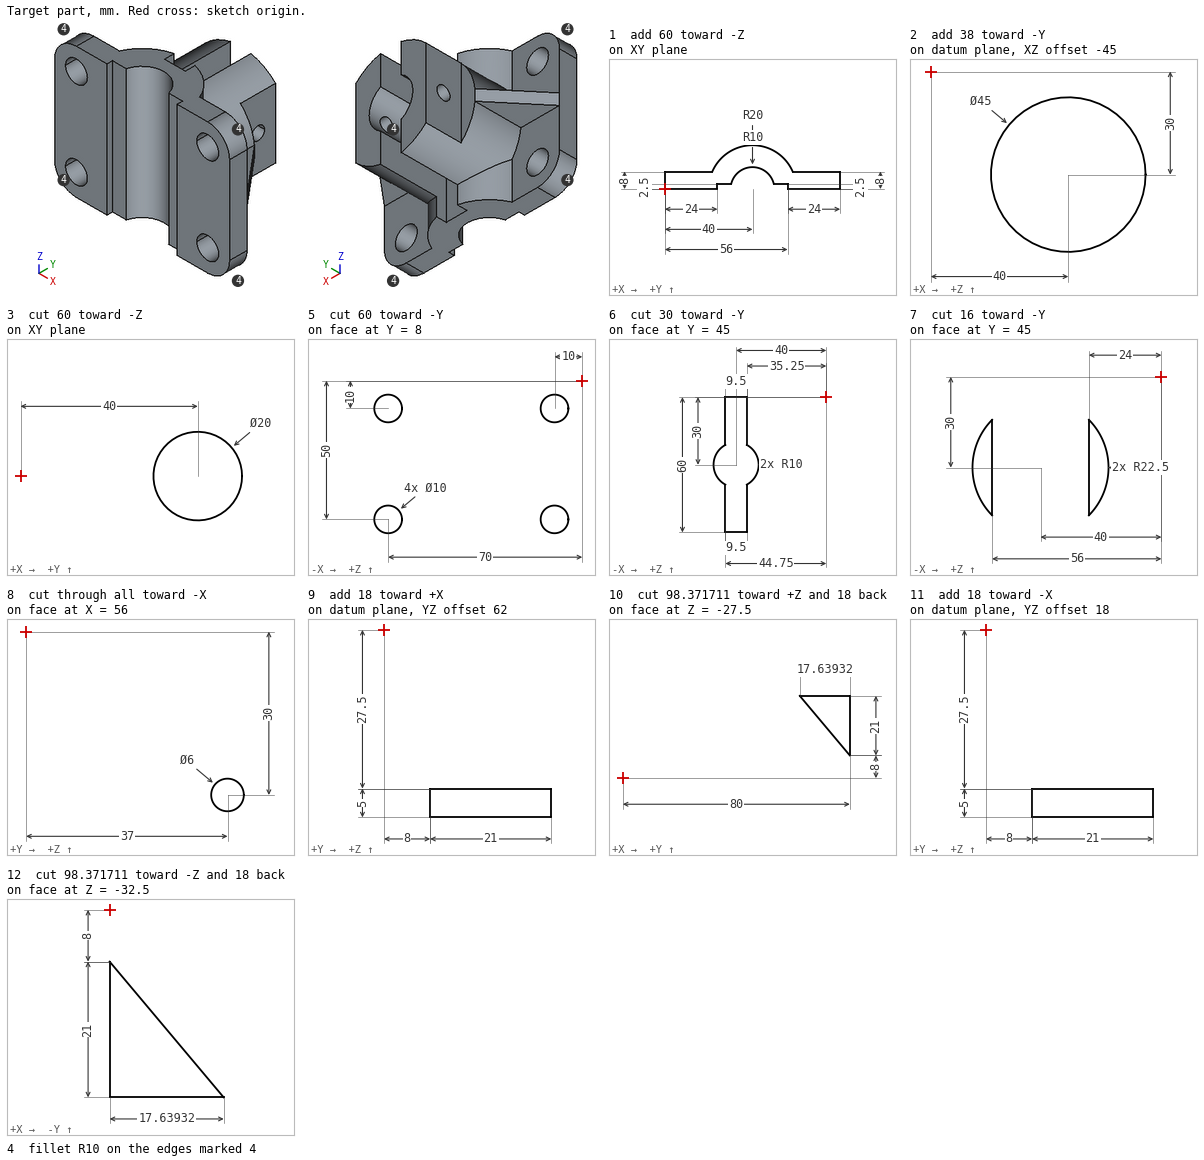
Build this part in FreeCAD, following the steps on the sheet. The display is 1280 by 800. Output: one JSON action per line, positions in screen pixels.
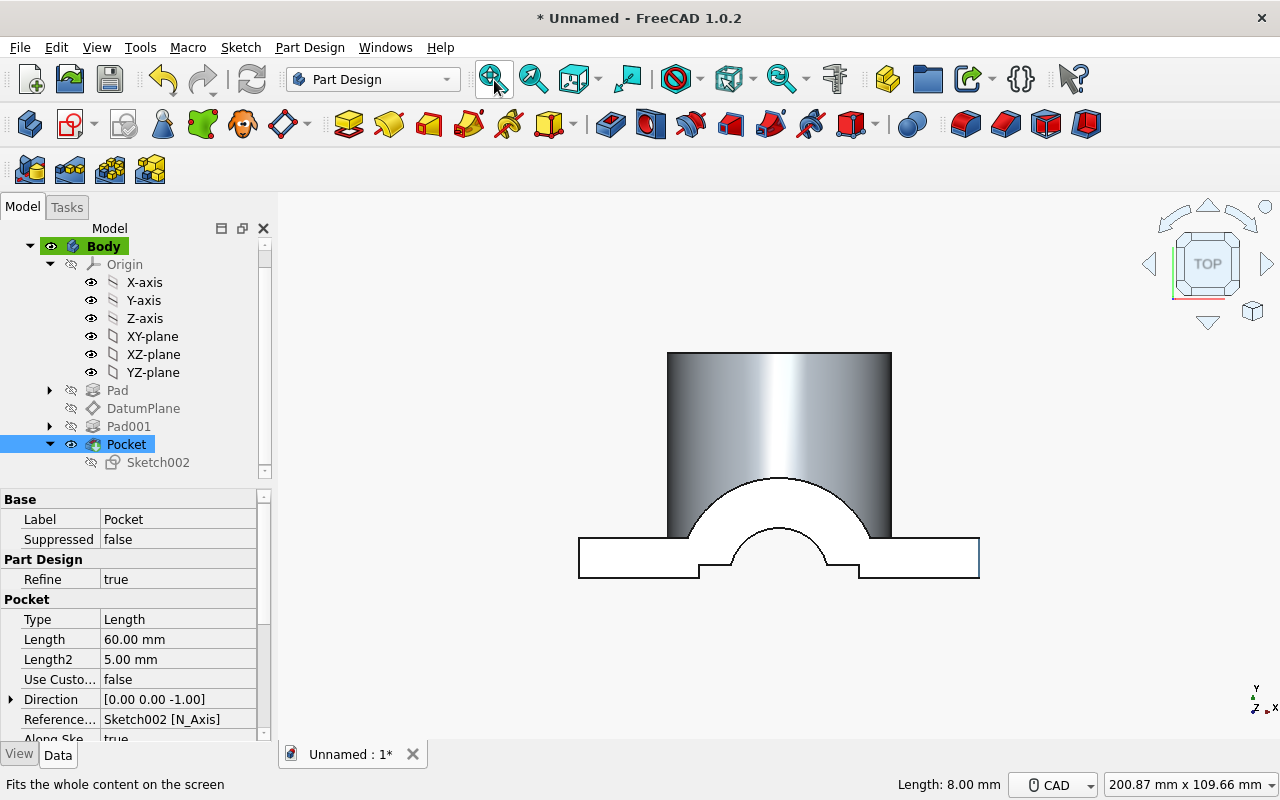
{"action": "left_click", "coordinate": [579, 557], "text": "ctrl"}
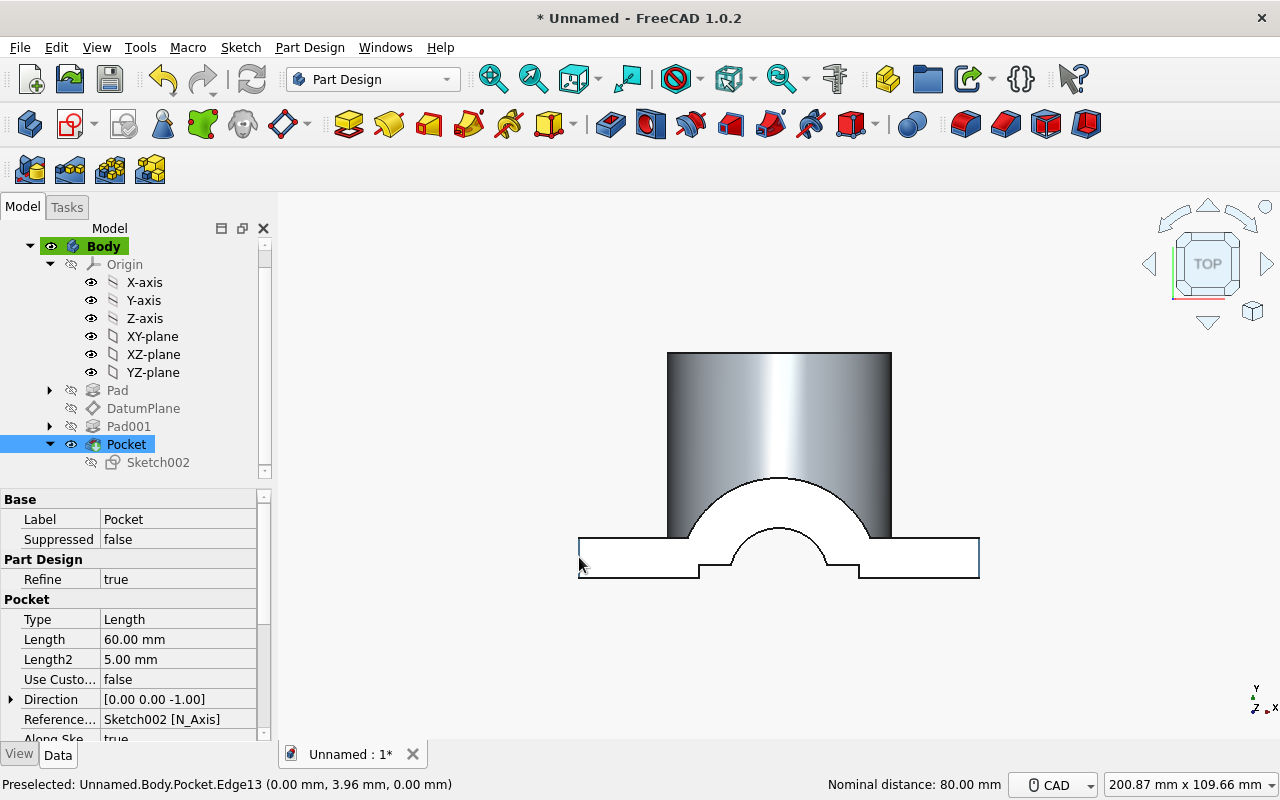
{"action": "key", "text": "1"}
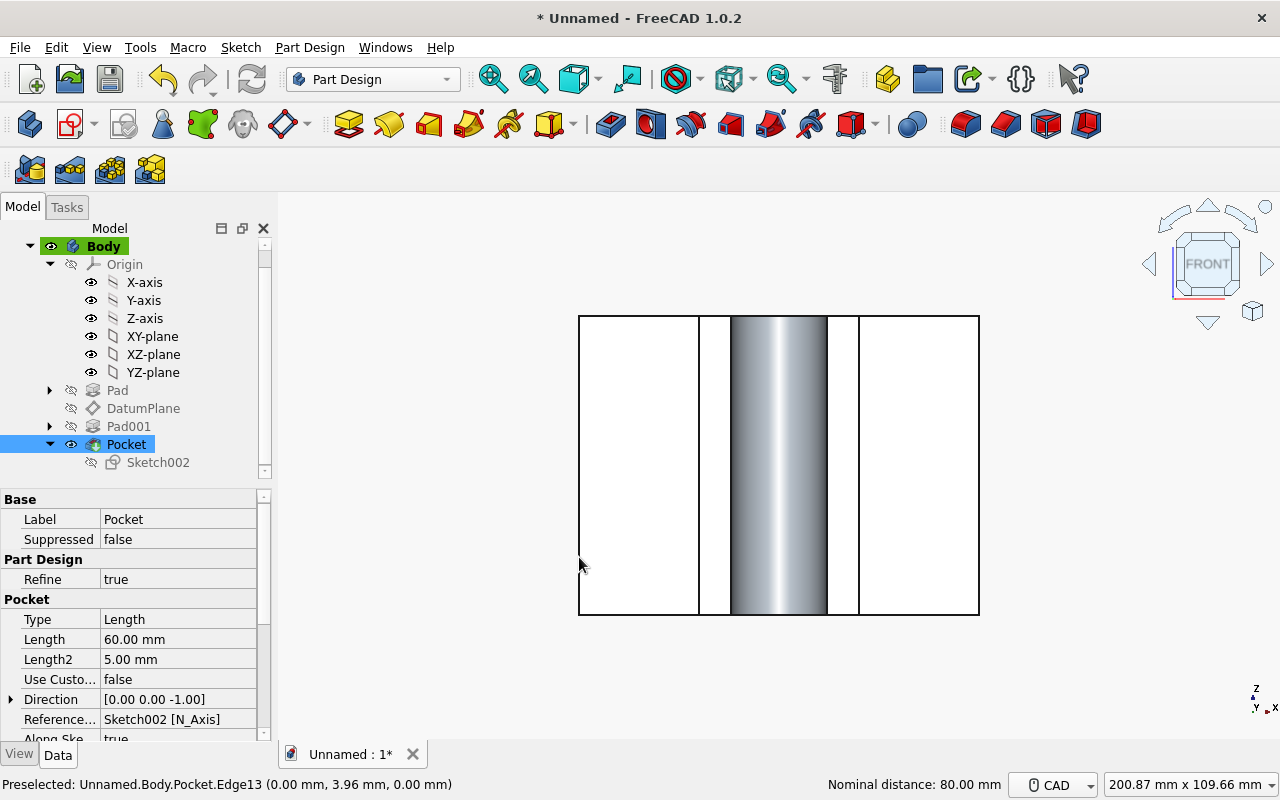
{"action": "key", "text": "3"}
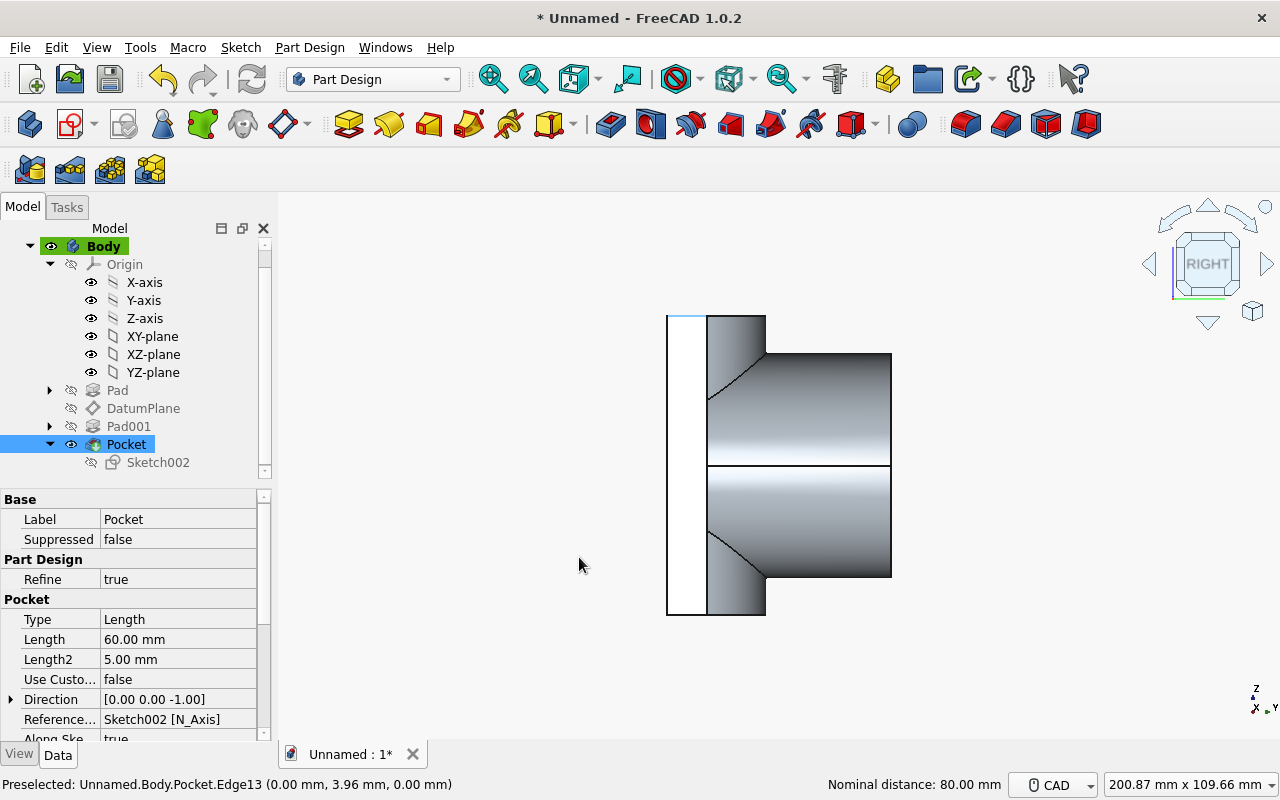
{"action": "left_click", "coordinate": [687, 614], "text": "ctrl"}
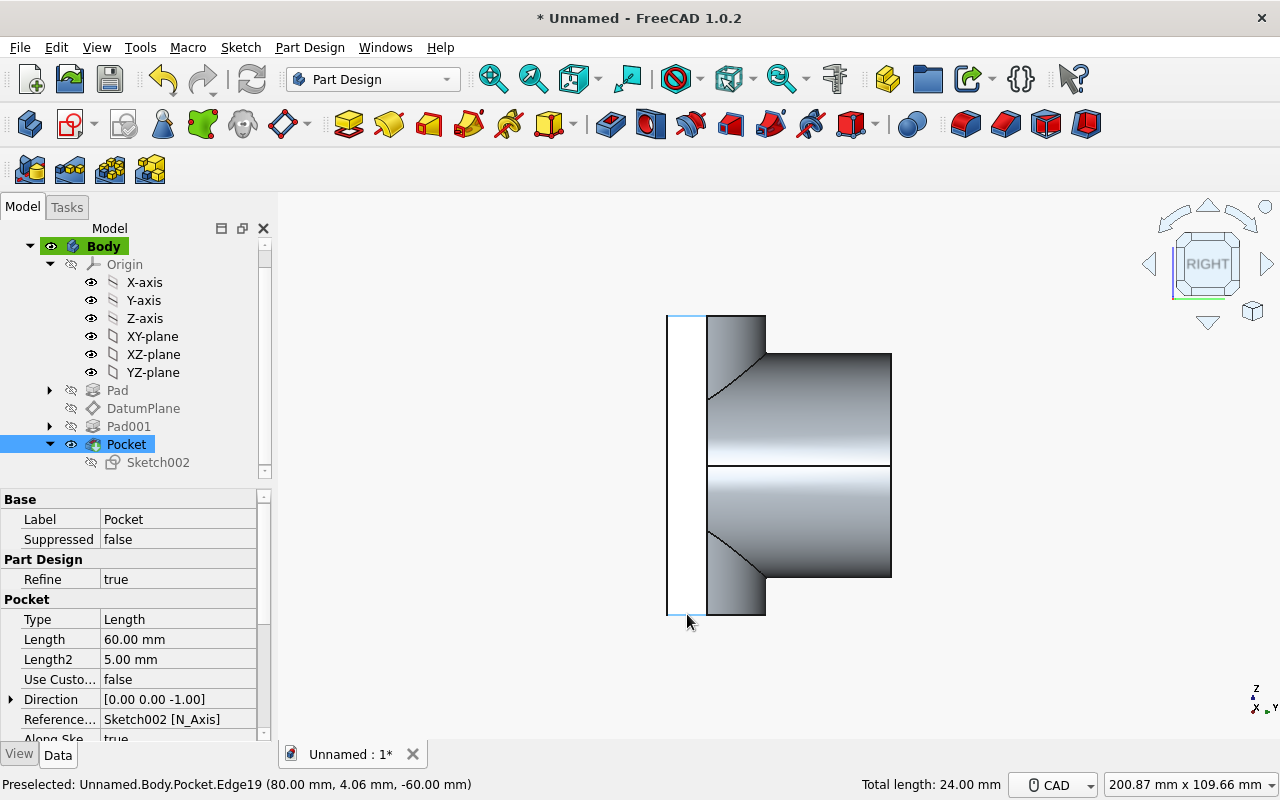
{"action": "key", "text": "5"}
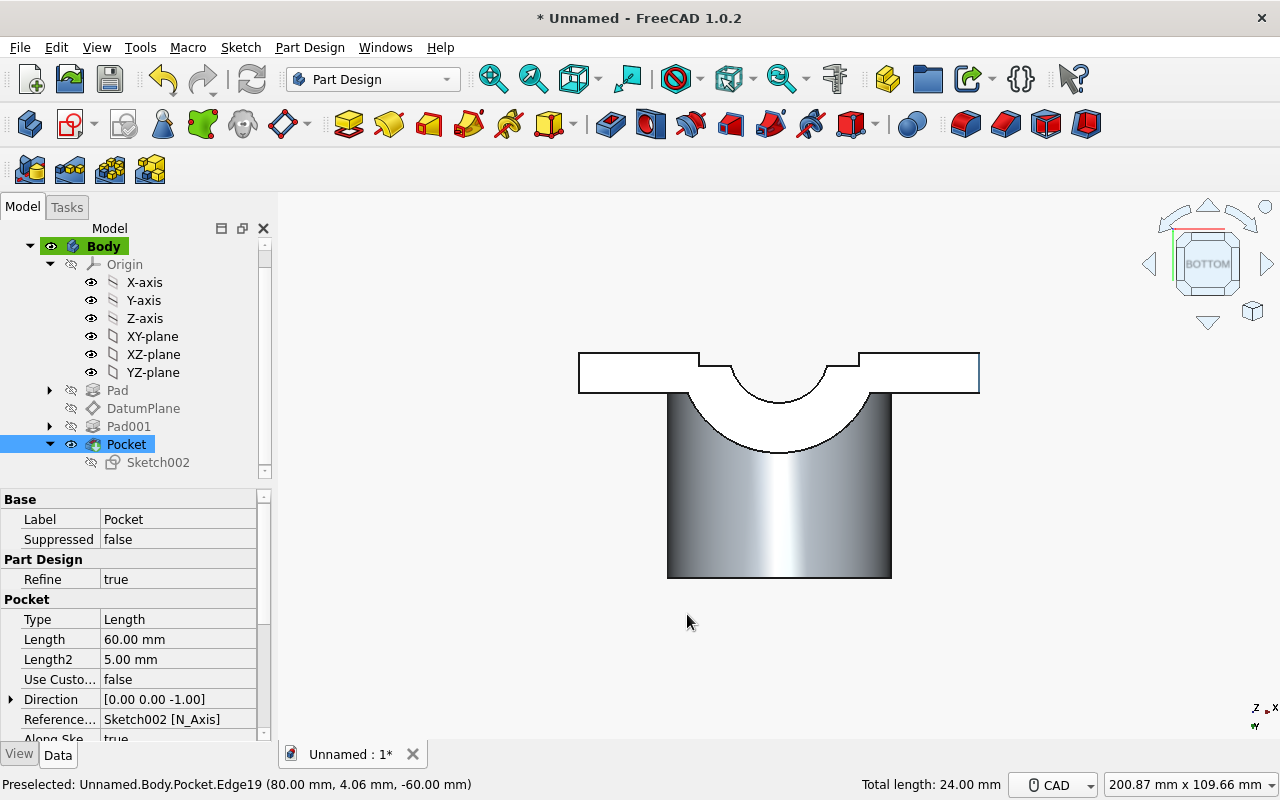
{"action": "left_click", "coordinate": [494, 80]}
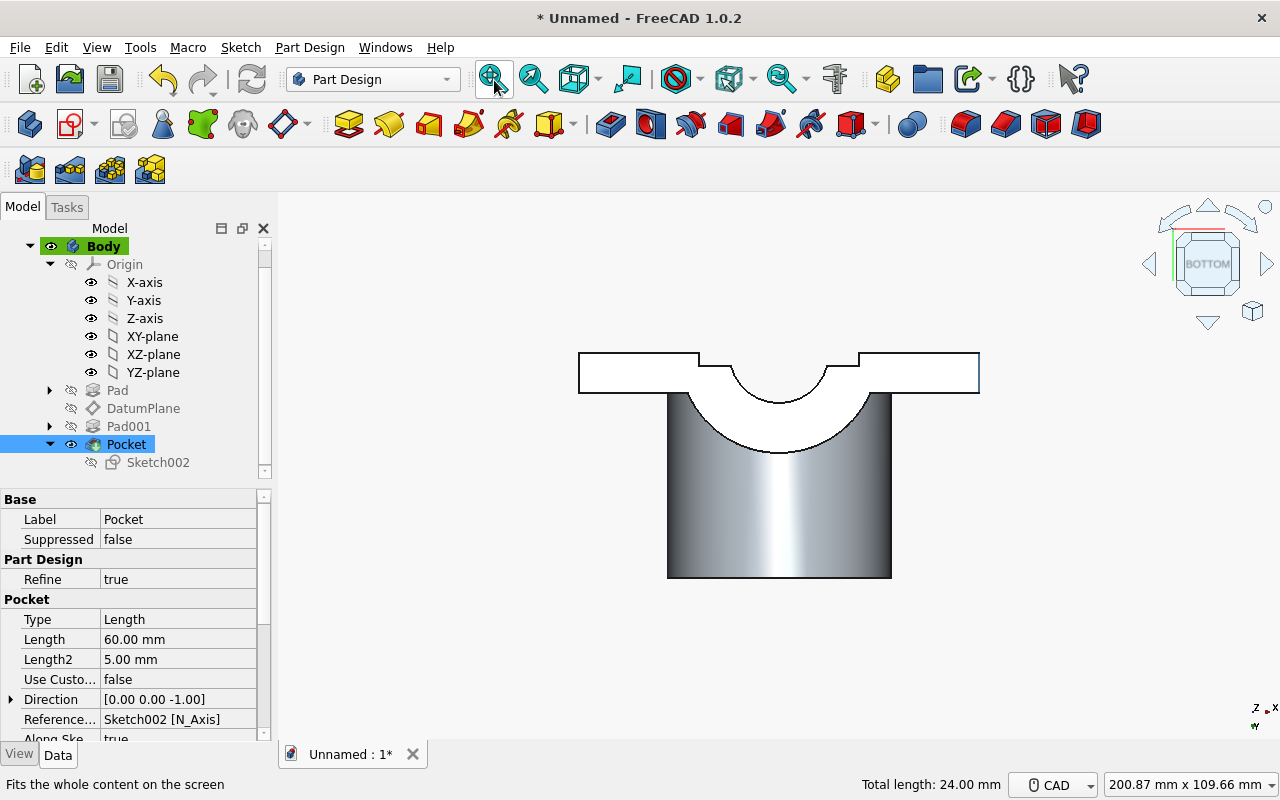
{"action": "left_click", "coordinate": [579, 372], "text": "ctrl"}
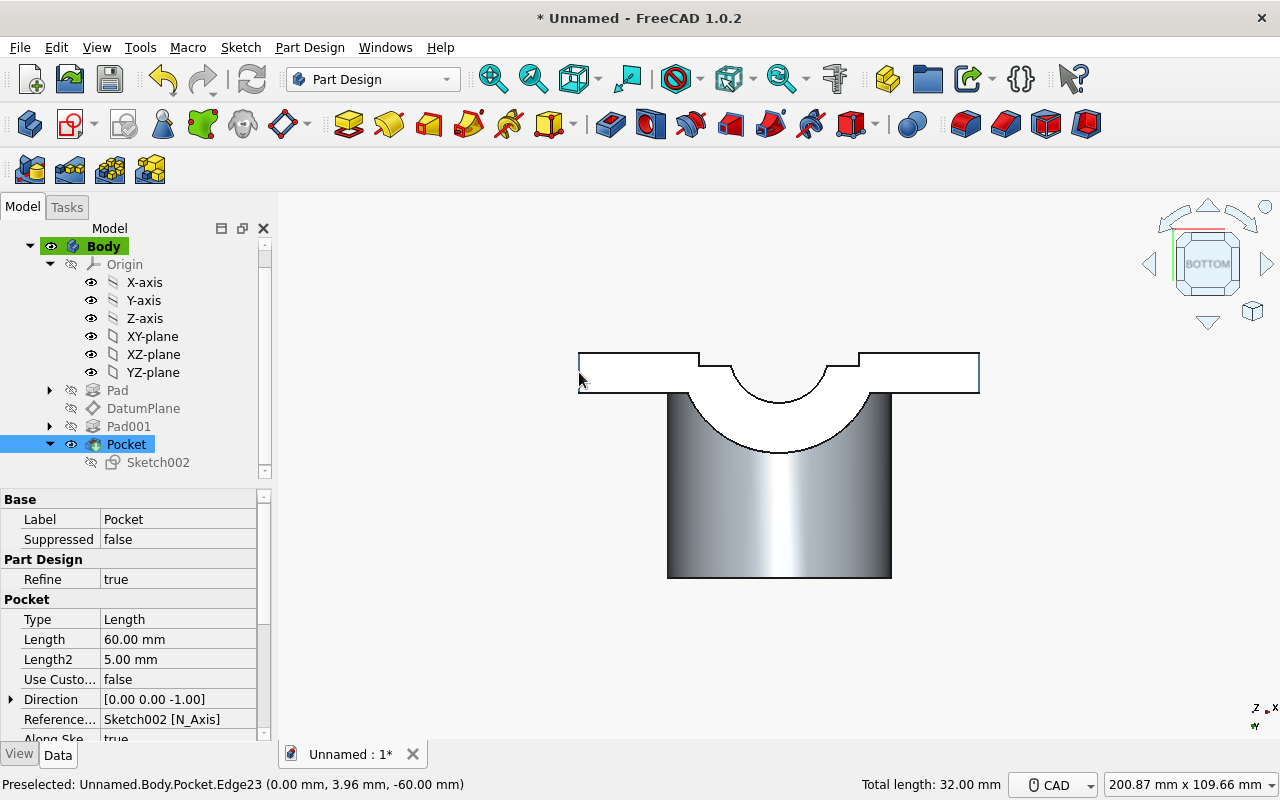
{"action": "left_click", "coordinate": [966, 124]}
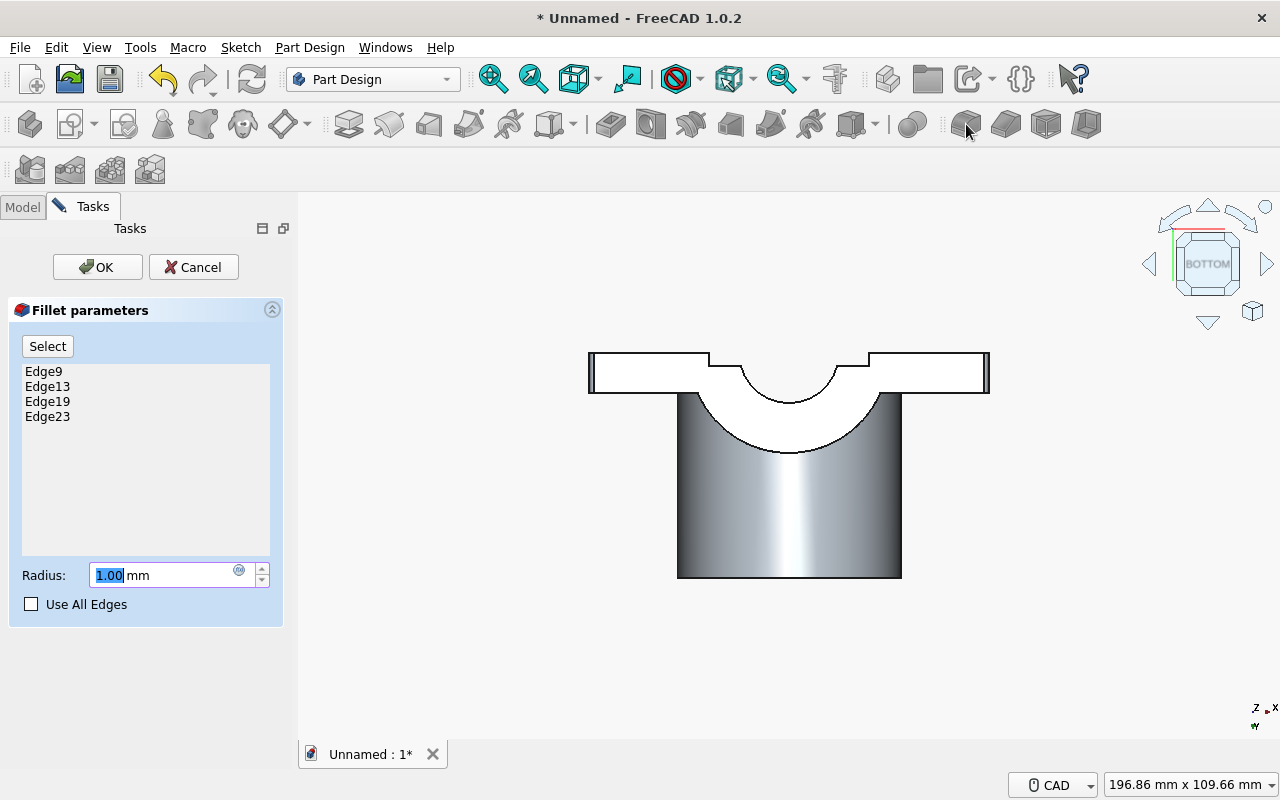
{"action": "type", "text": "10"}
{"action": "key", "text": "Tab"}